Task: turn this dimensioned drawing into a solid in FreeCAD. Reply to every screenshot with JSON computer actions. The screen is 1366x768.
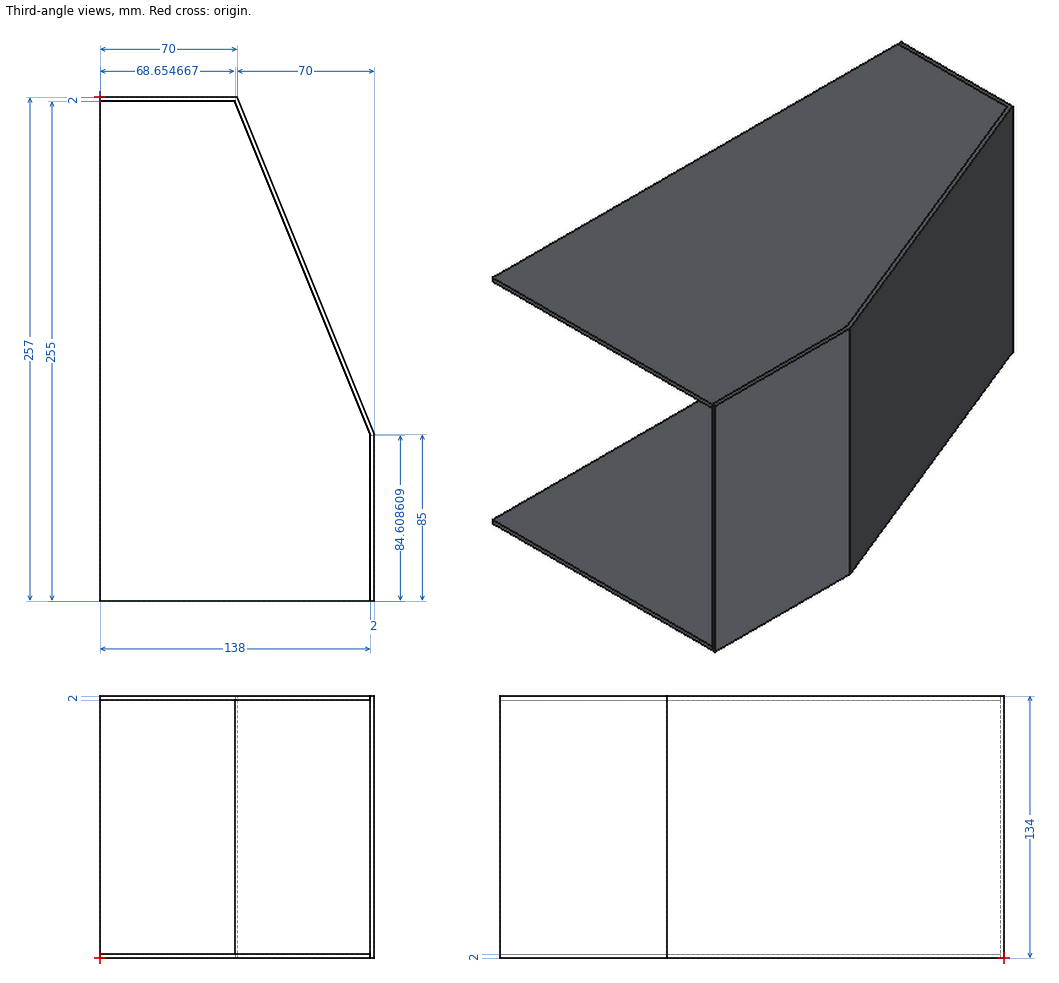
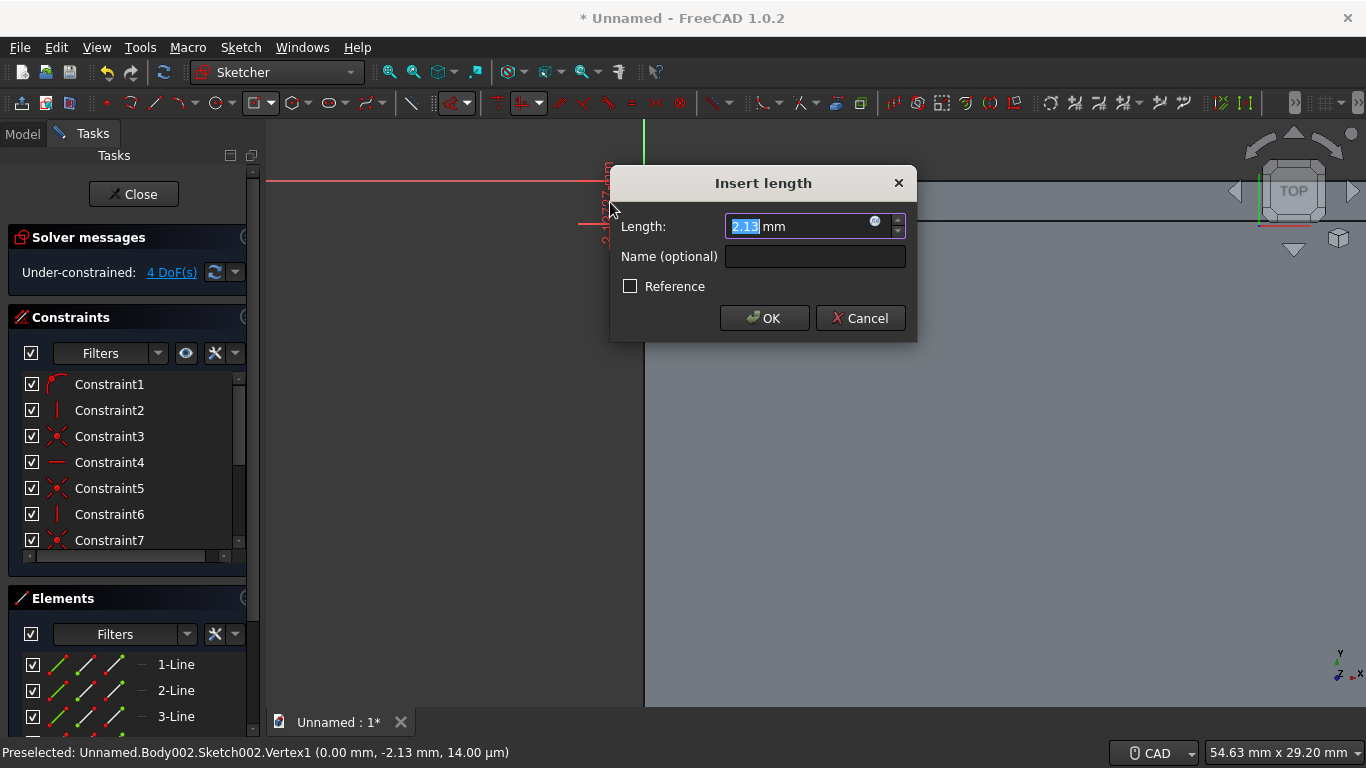
{"action": "type", "text": "2"}
{"action": "key", "text": "Return"}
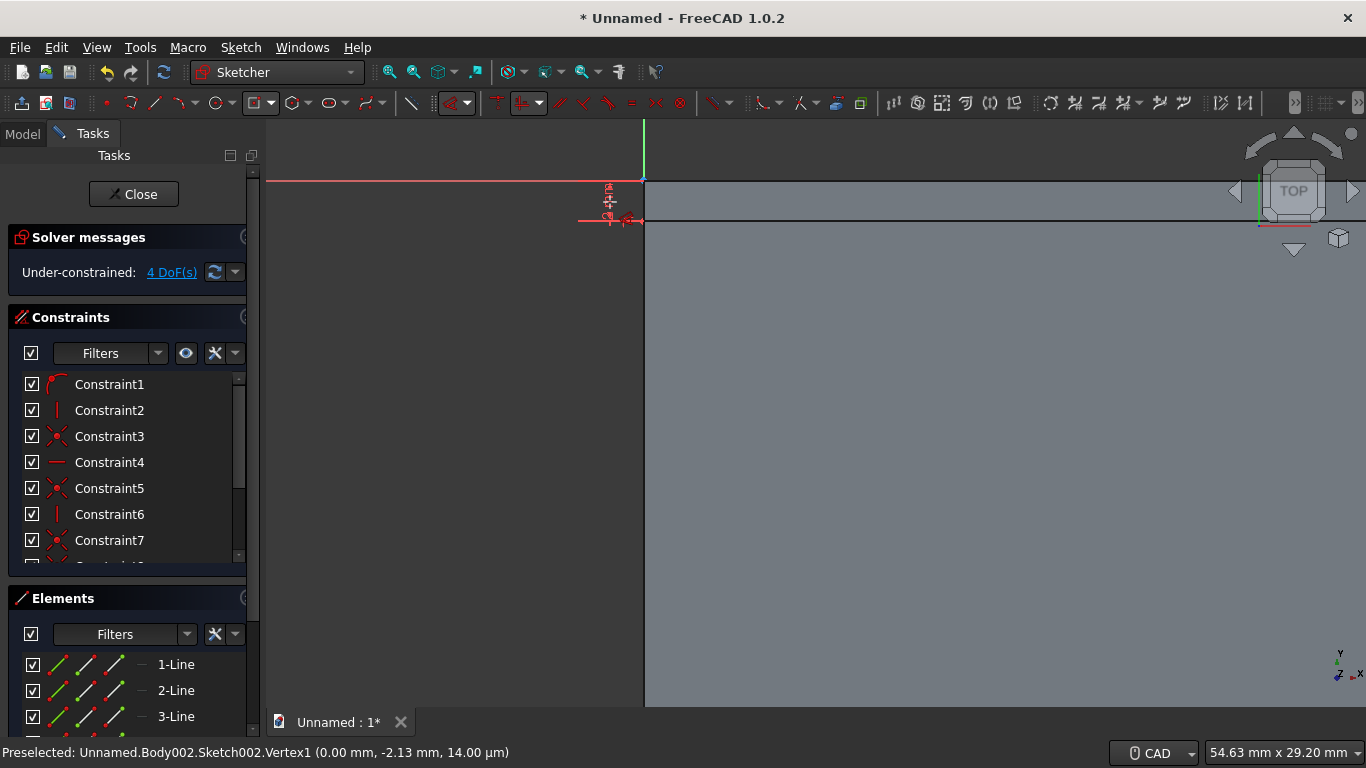
{"action": "scroll", "coordinate": [644, 224], "scroll_direction": "down", "scroll_amount": 13}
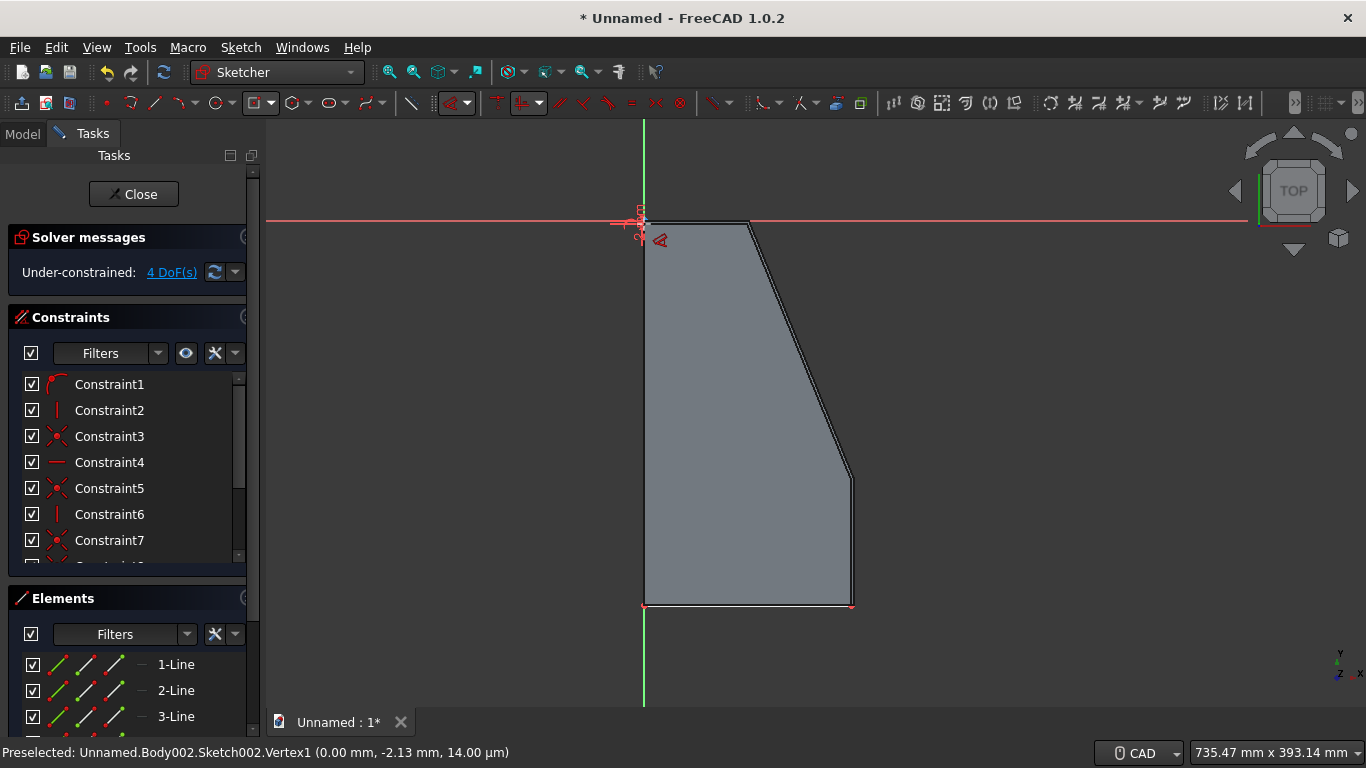
{"action": "left_click", "coordinate": [644, 339]}
{"action": "left_click", "coordinate": [610, 415]}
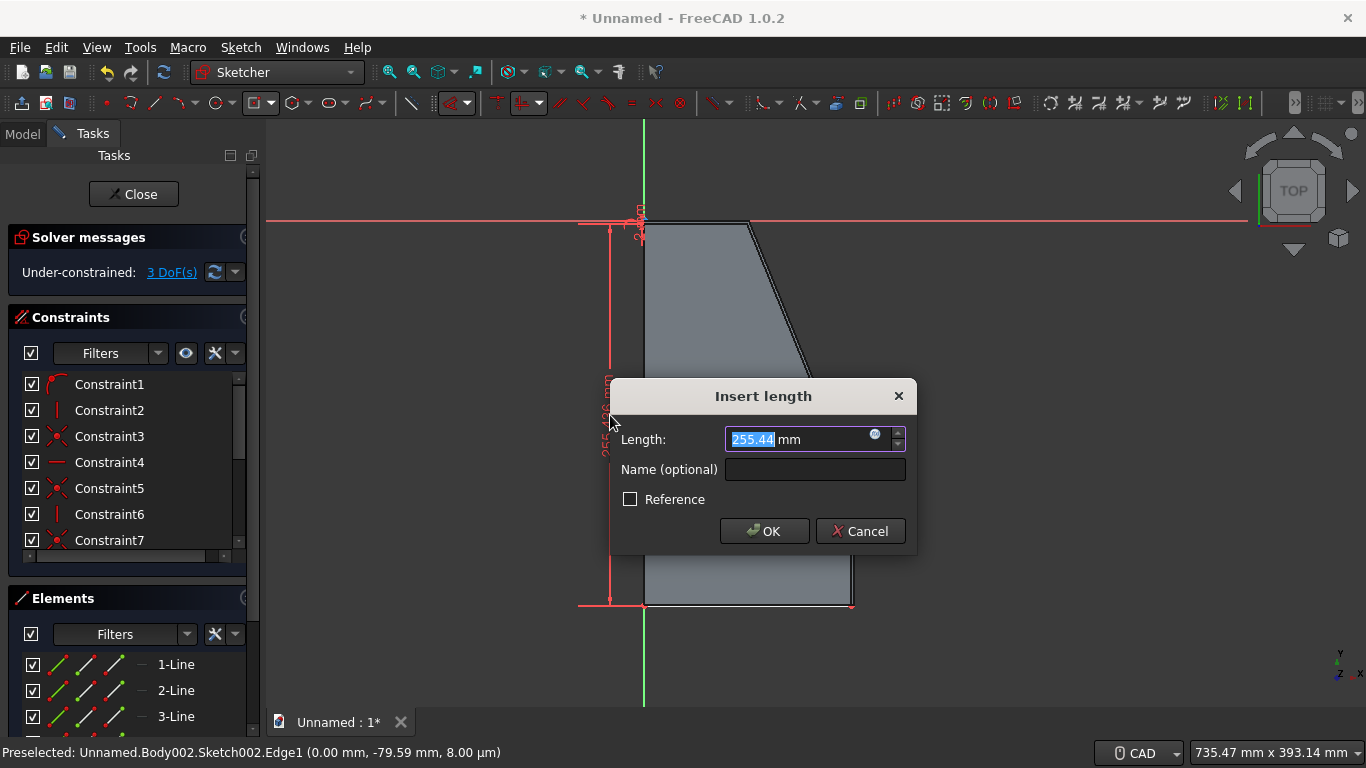
{"action": "type", "text": "255"}
{"action": "key", "text": "Return"}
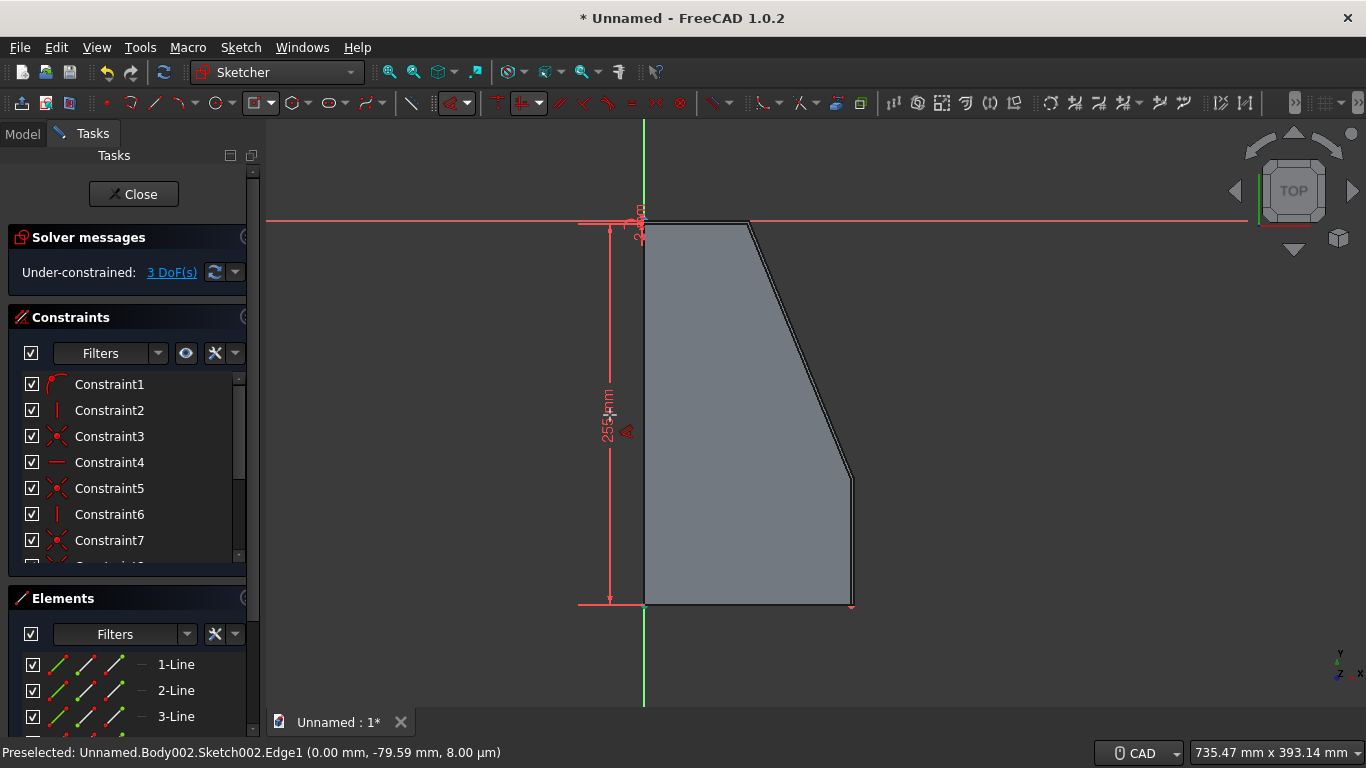
{"action": "left_click", "coordinate": [706, 605]}
{"action": "left_click", "coordinate": [748, 639]}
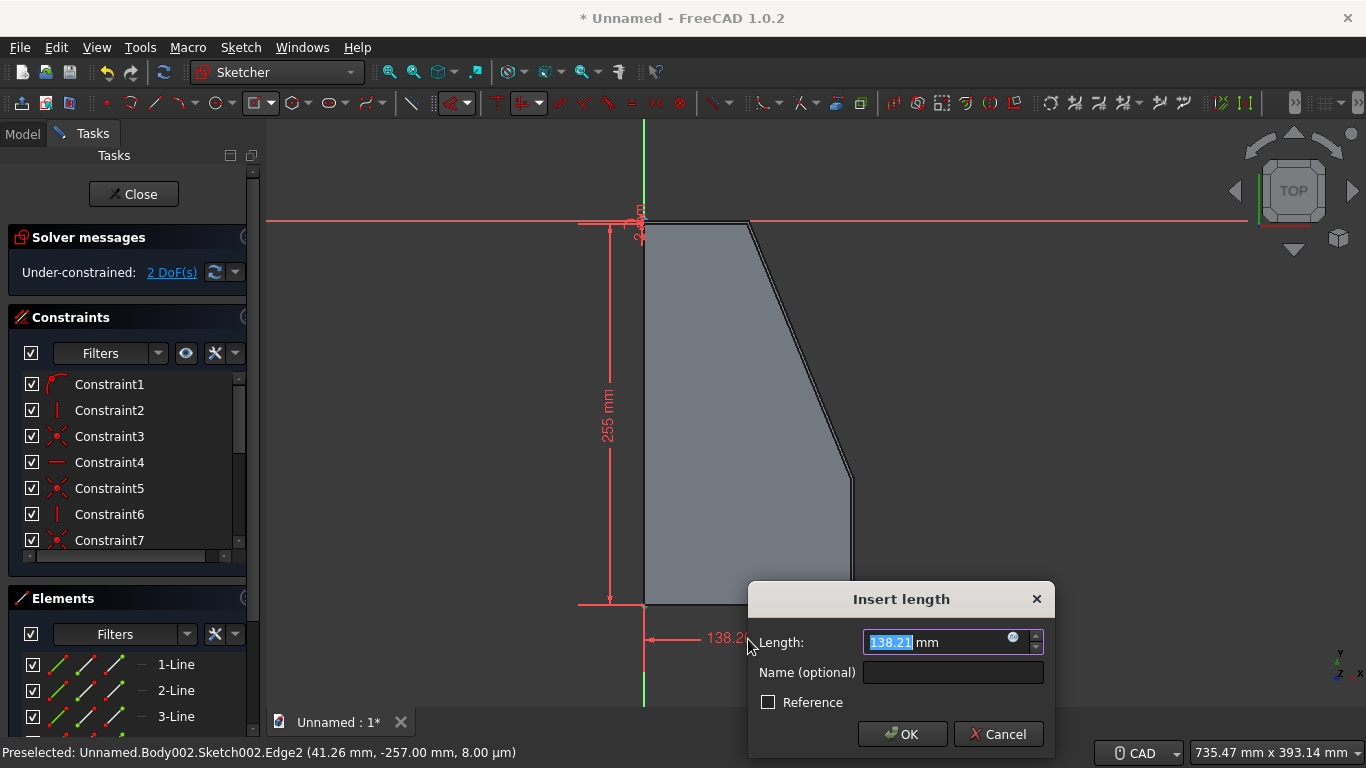
{"action": "type", "text": "138"}
{"action": "key", "text": "Return"}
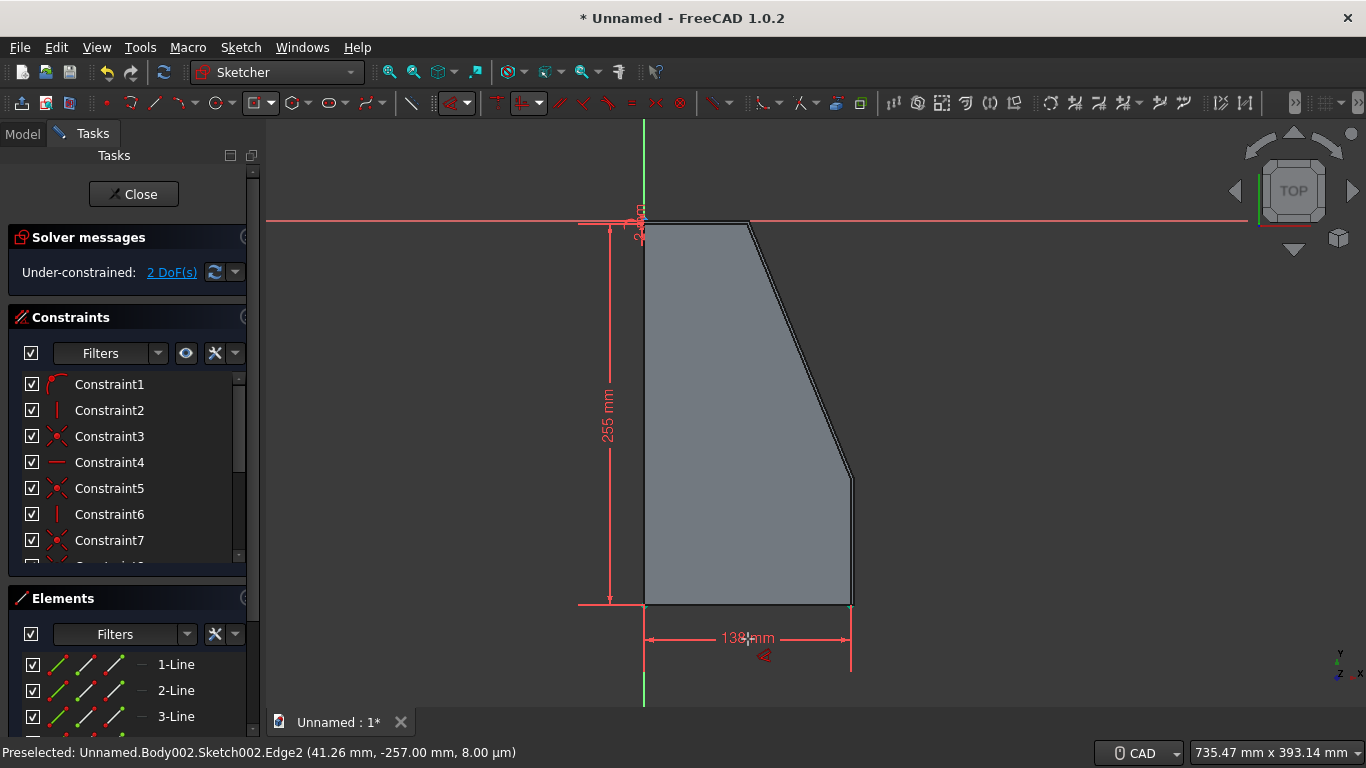
{"action": "left_click", "coordinate": [851, 568]}
{"action": "left_click", "coordinate": [885, 543]}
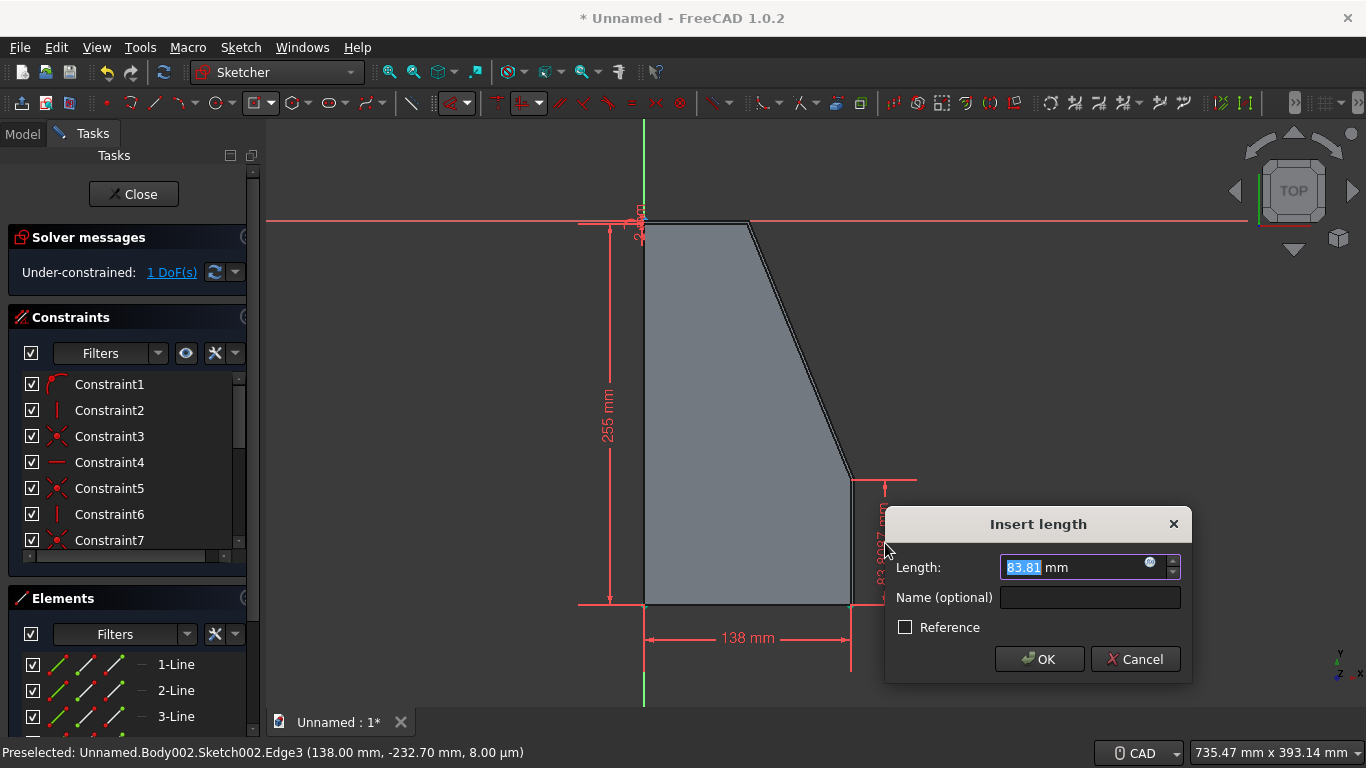
{"action": "type", "text": "84.608609"}
{"action": "key", "text": "Return"}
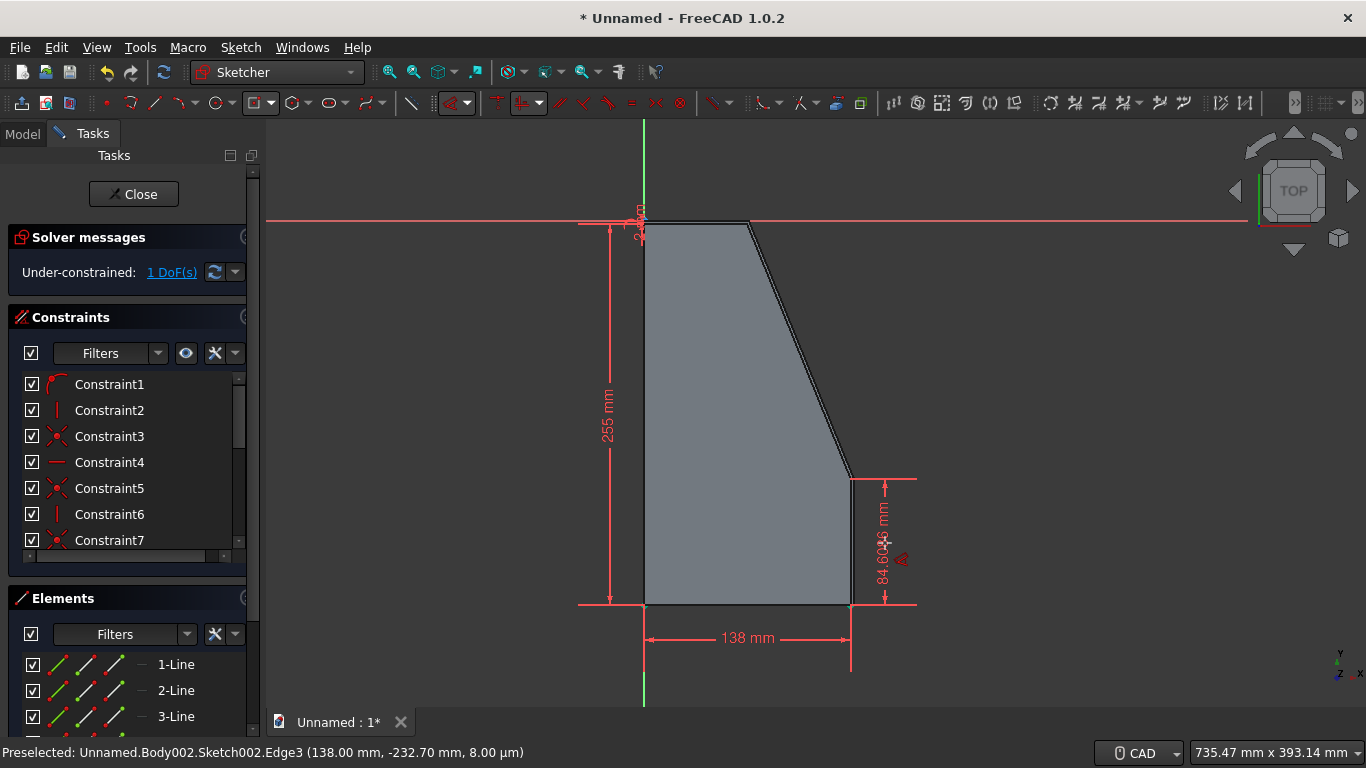
{"action": "left_click", "coordinate": [716, 224]}
{"action": "left_click", "coordinate": [696, 190]}